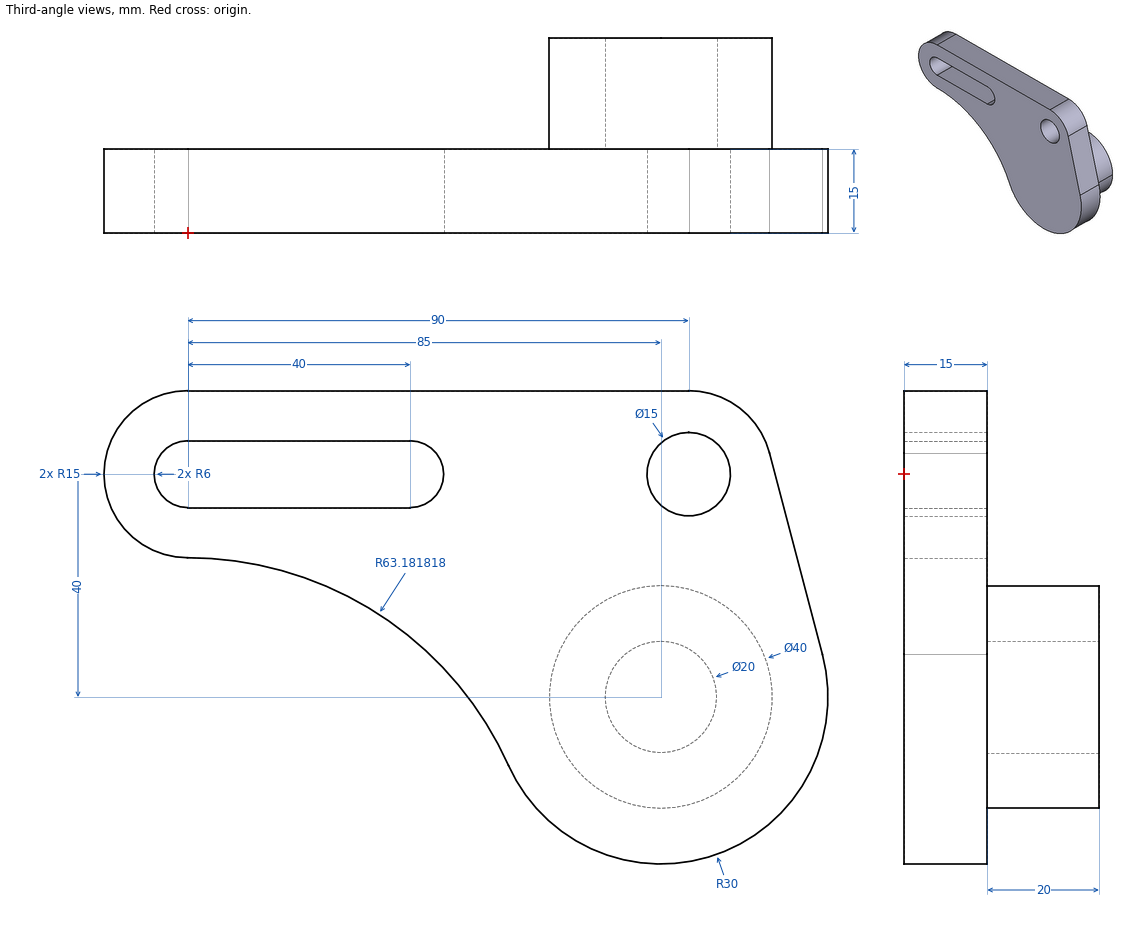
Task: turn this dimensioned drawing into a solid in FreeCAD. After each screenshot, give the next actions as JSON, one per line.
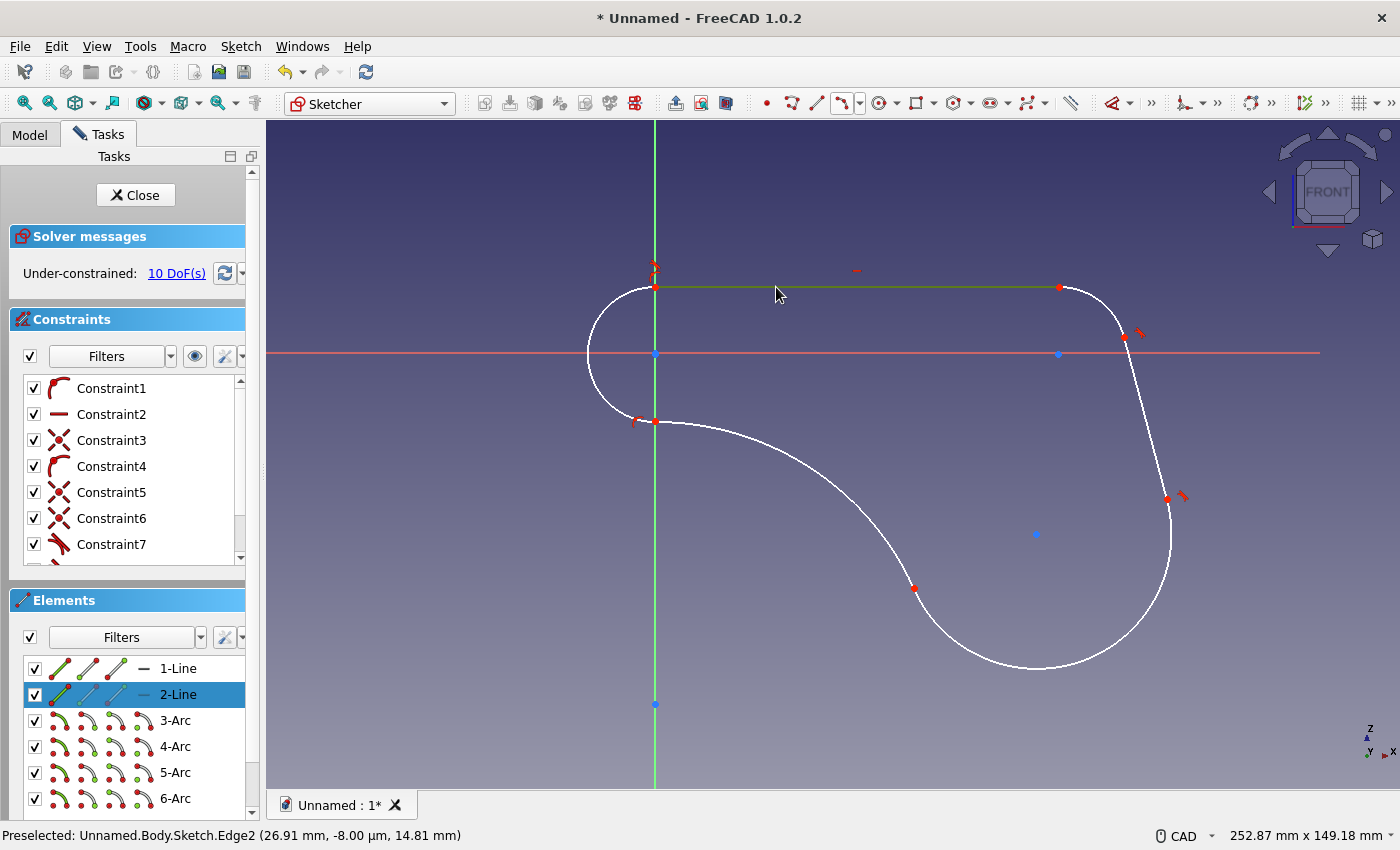
{"action": "left_click", "coordinate": [1112, 314]}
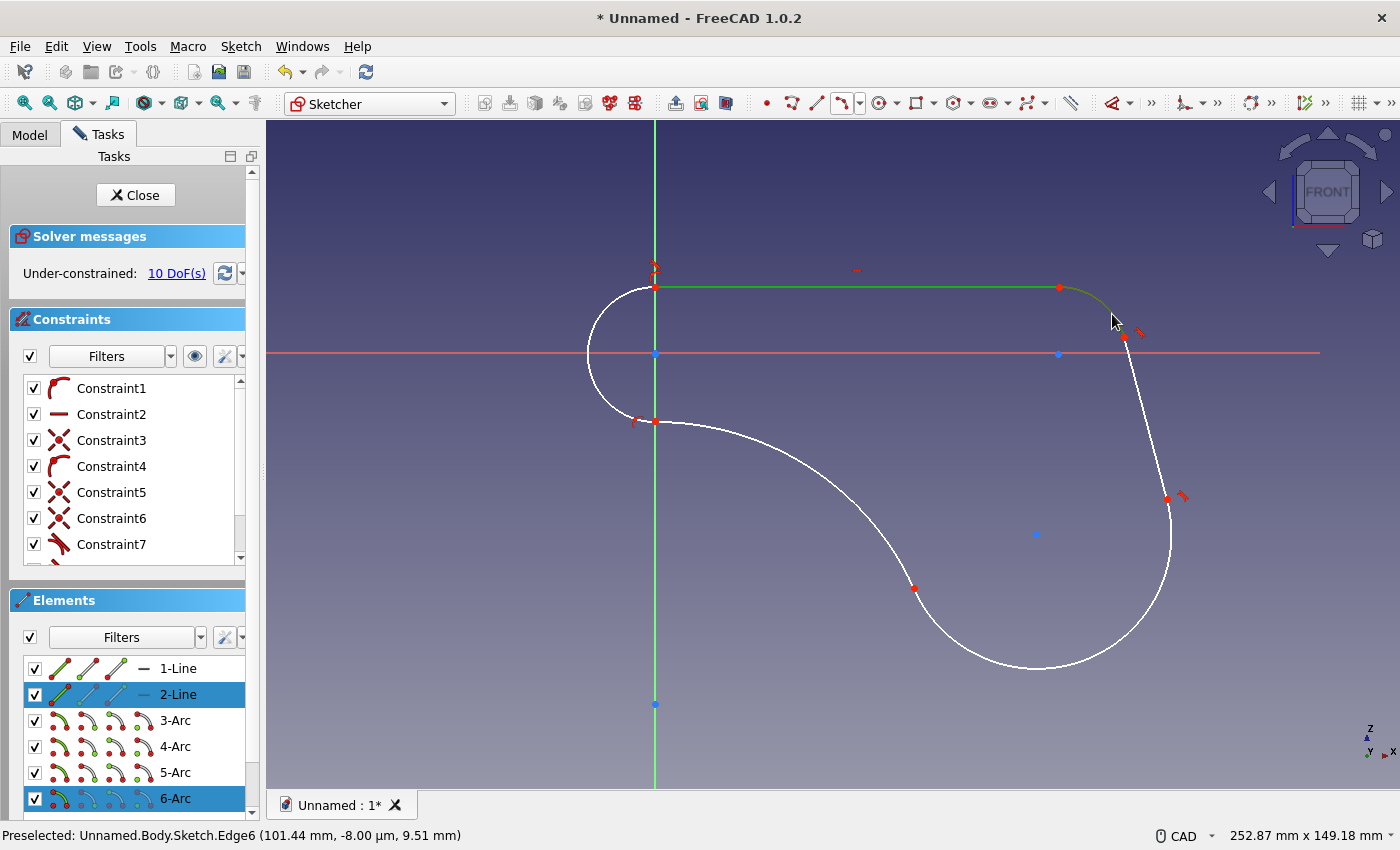
{"action": "key", "text": "t"}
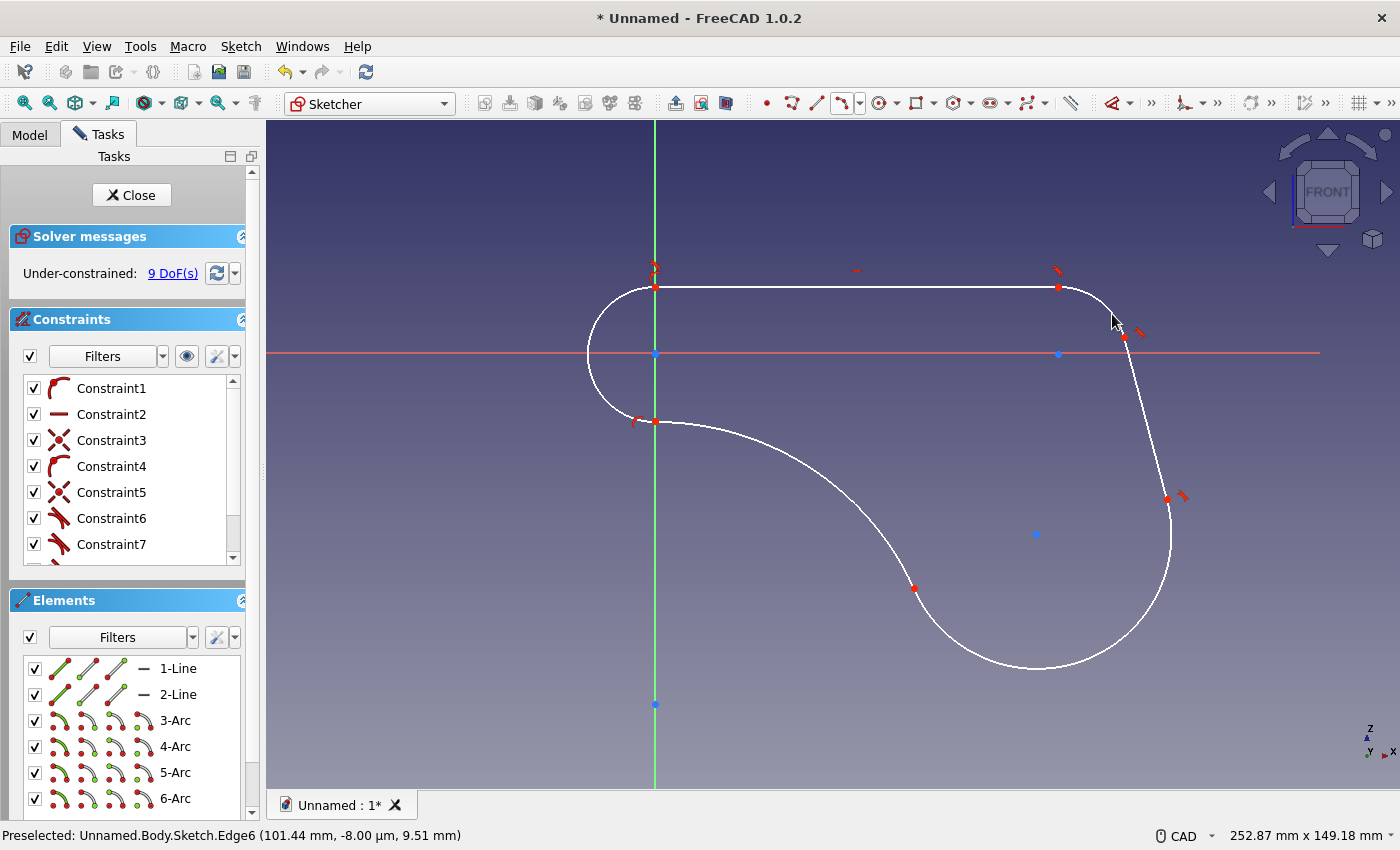
{"action": "left_click", "coordinate": [1003, 664]}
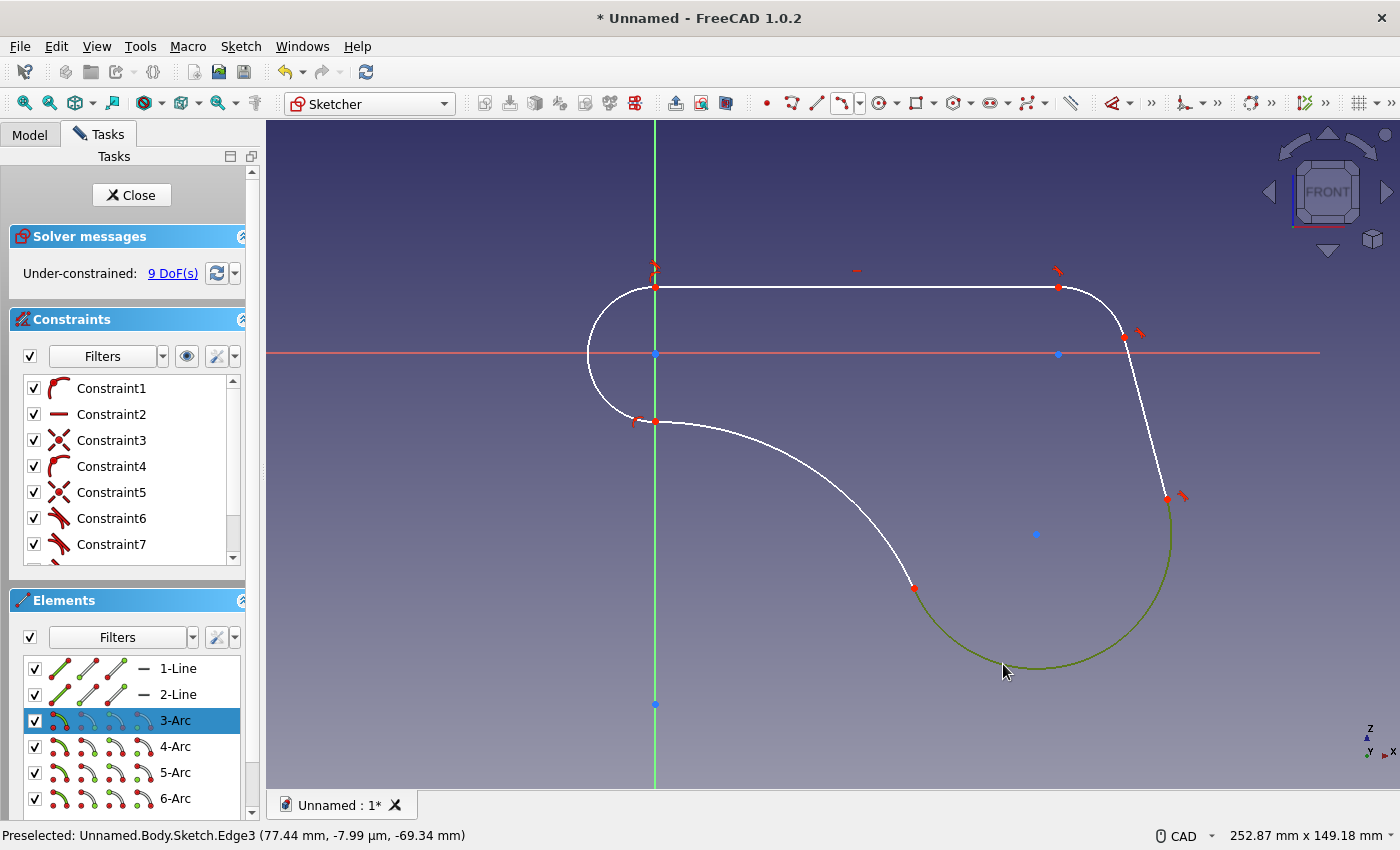
{"action": "left_click", "coordinate": [860, 509]}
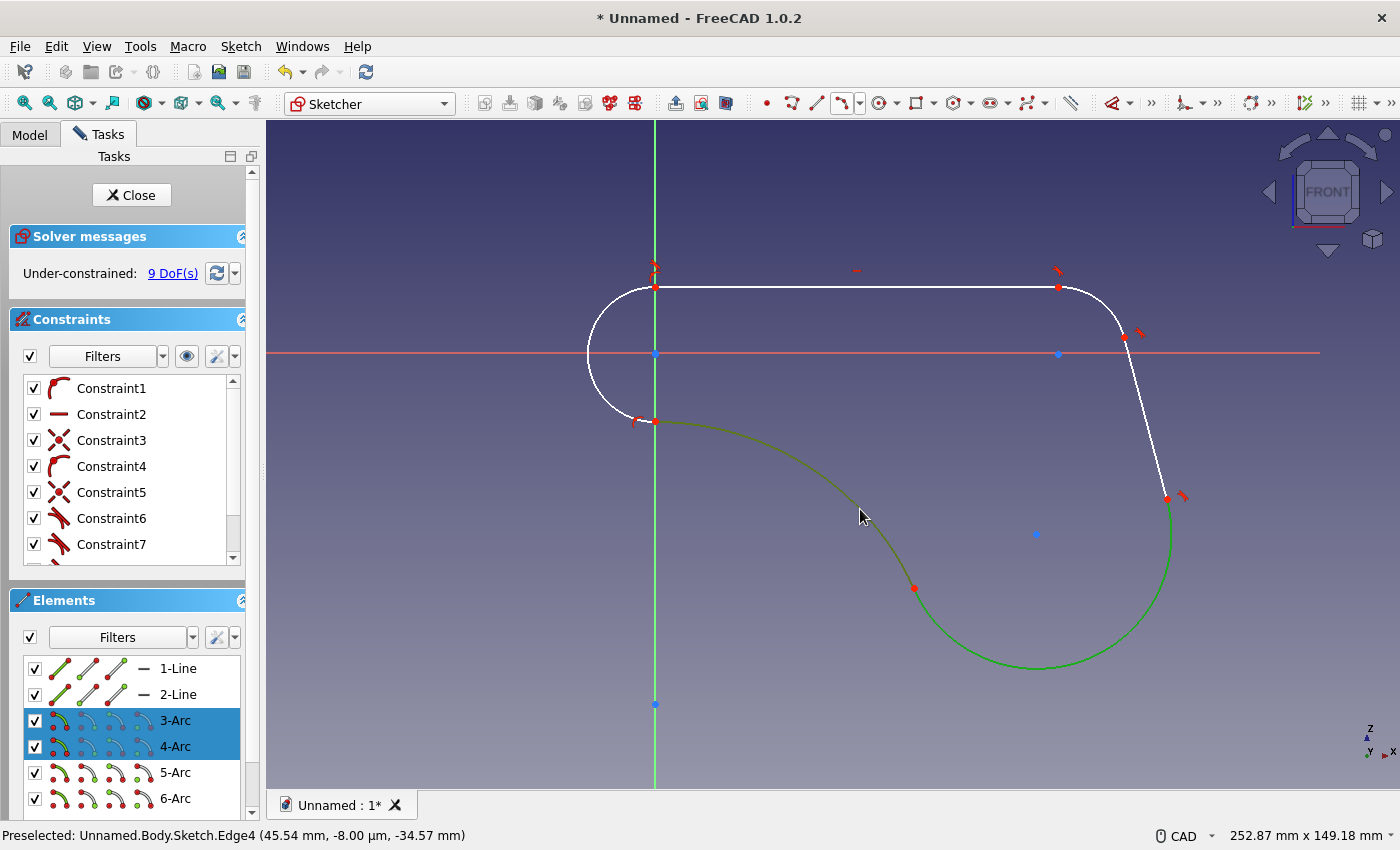
{"action": "key", "text": "t"}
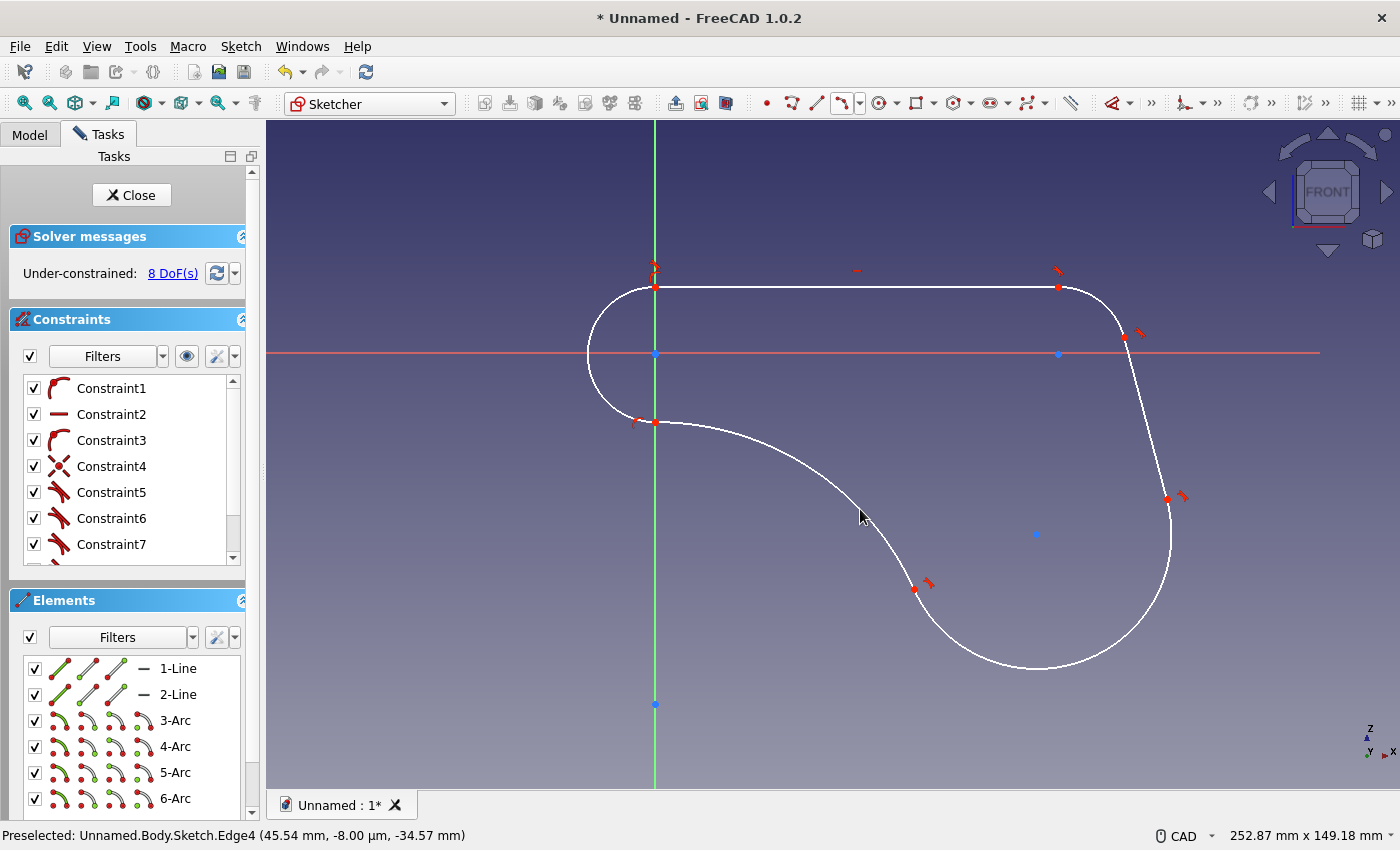
{"action": "left_click", "coordinate": [601, 315]}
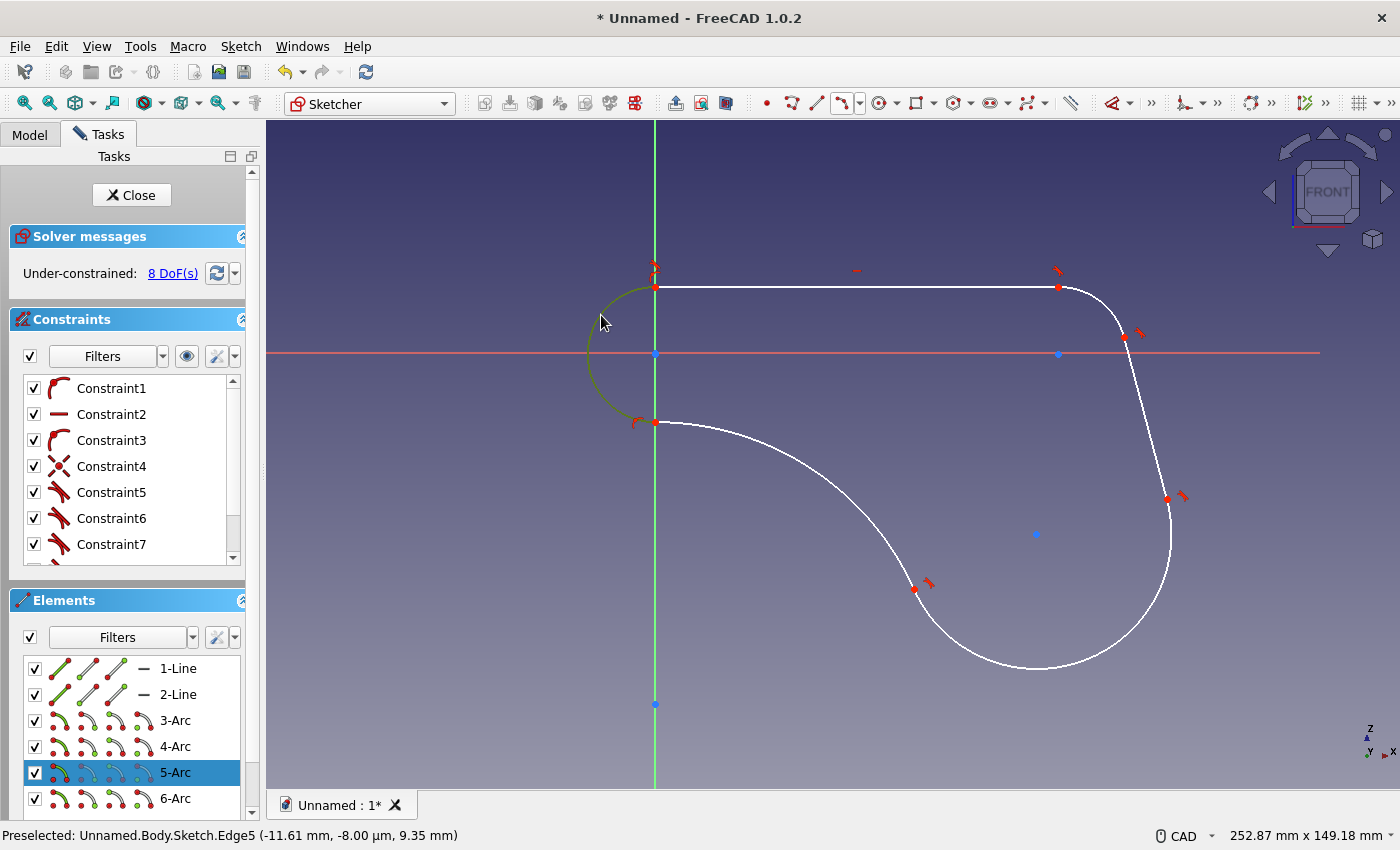
{"action": "left_click", "coordinate": [1112, 314]}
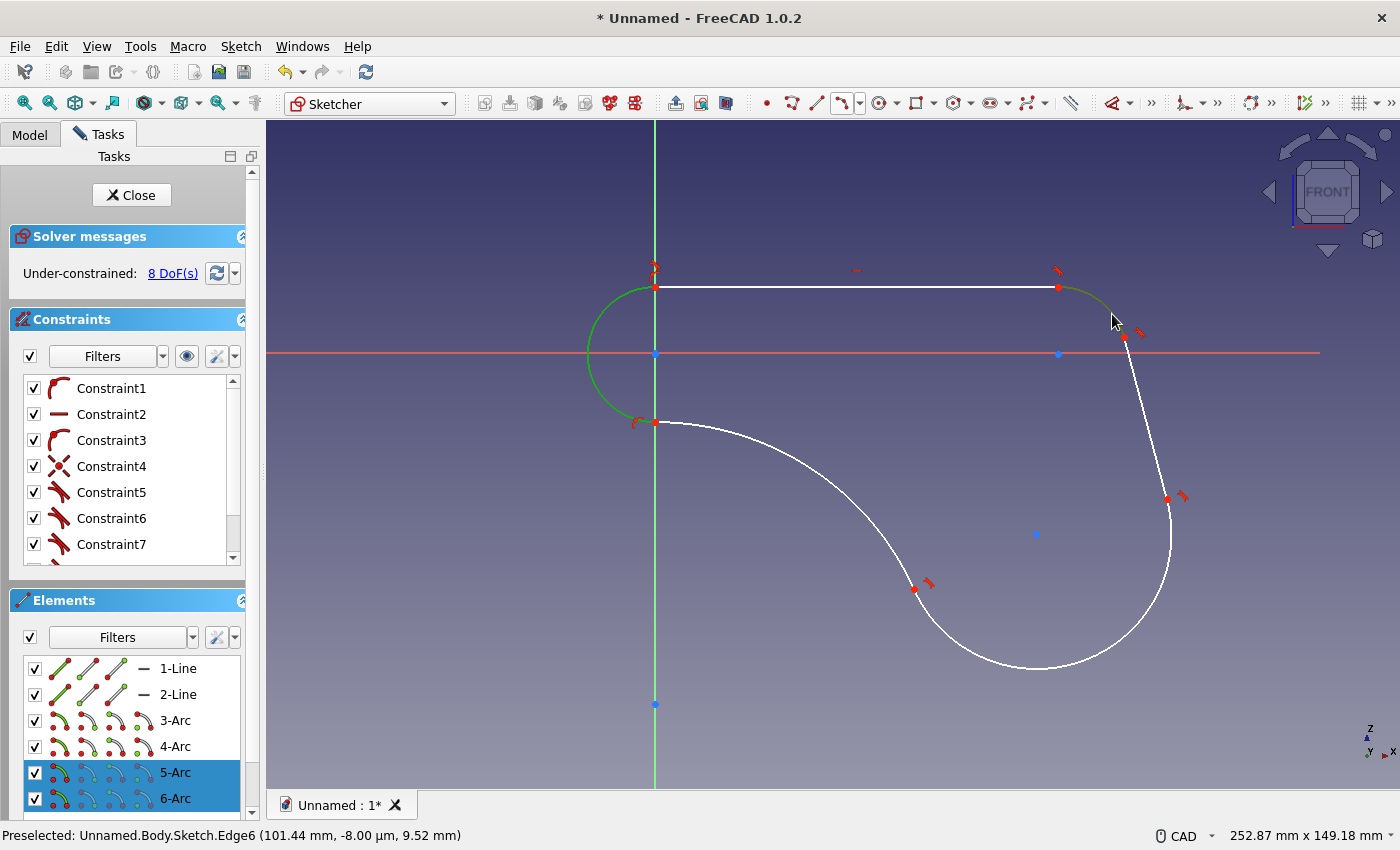
{"action": "key", "text": "e"}